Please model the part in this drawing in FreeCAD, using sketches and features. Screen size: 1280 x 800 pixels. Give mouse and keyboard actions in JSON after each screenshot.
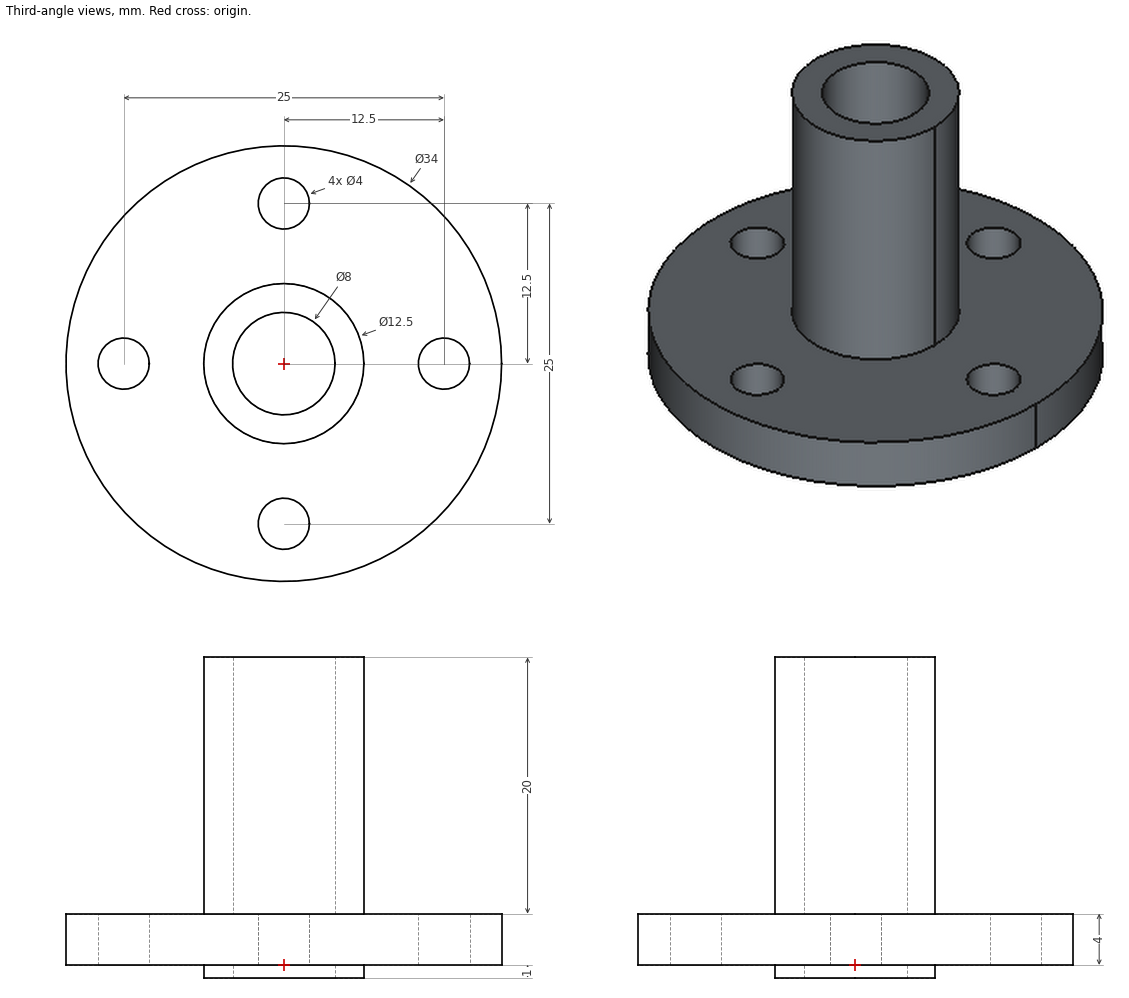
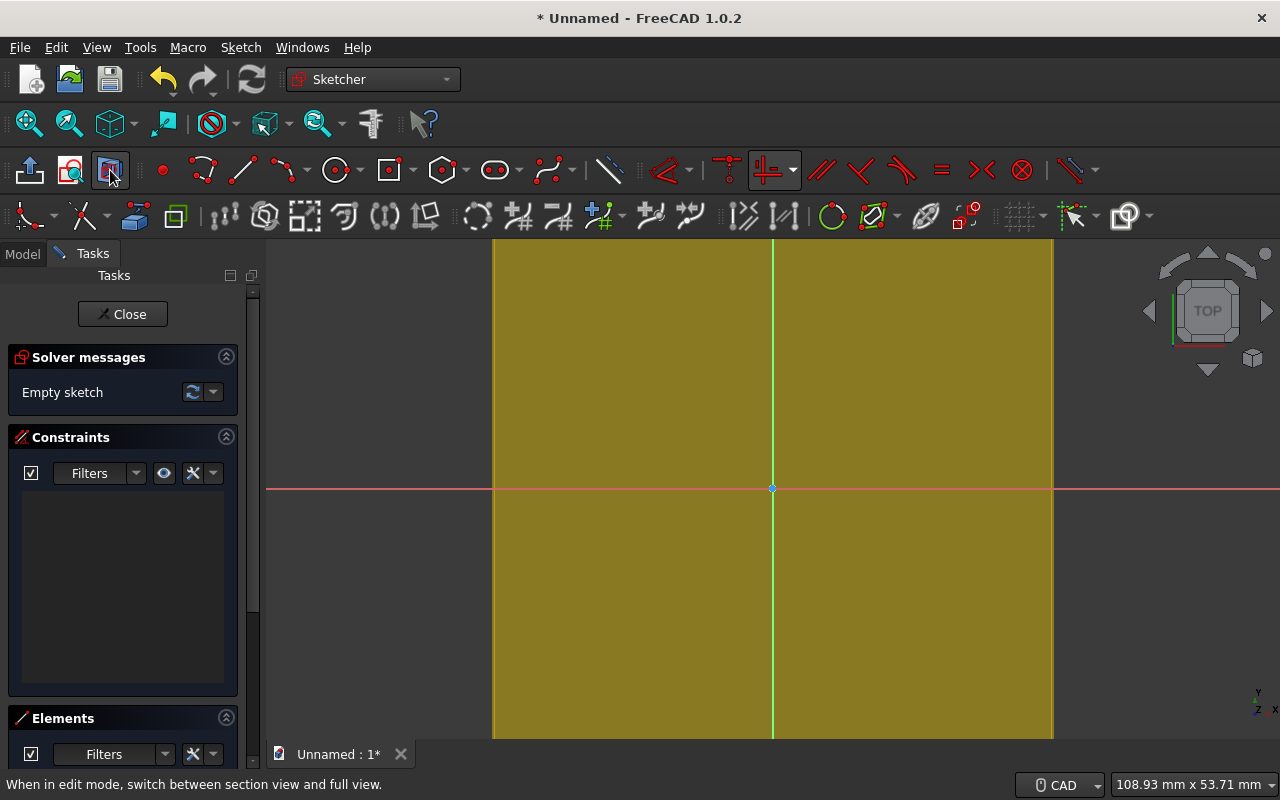
{"action": "scroll", "coordinate": [813, 489], "scroll_direction": "up", "scroll_amount": 5}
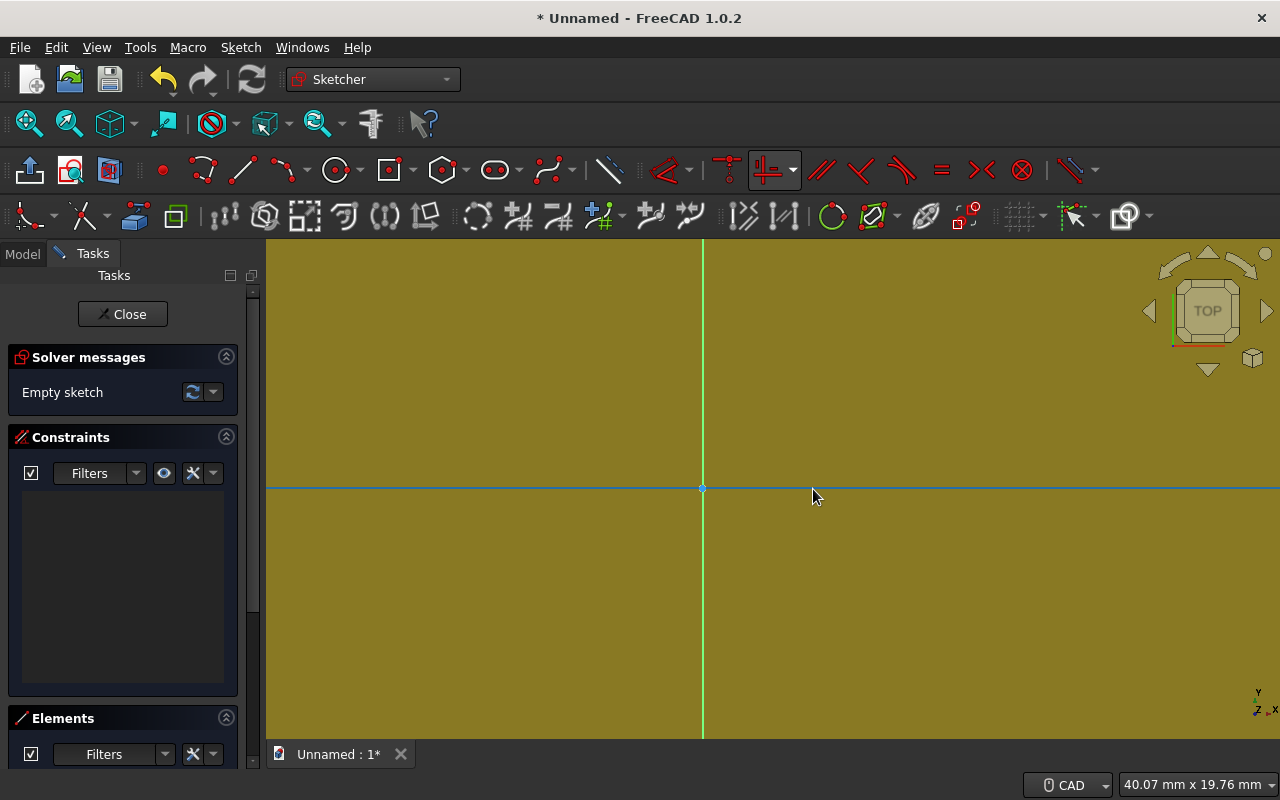
{"action": "left_click", "coordinate": [336, 170]}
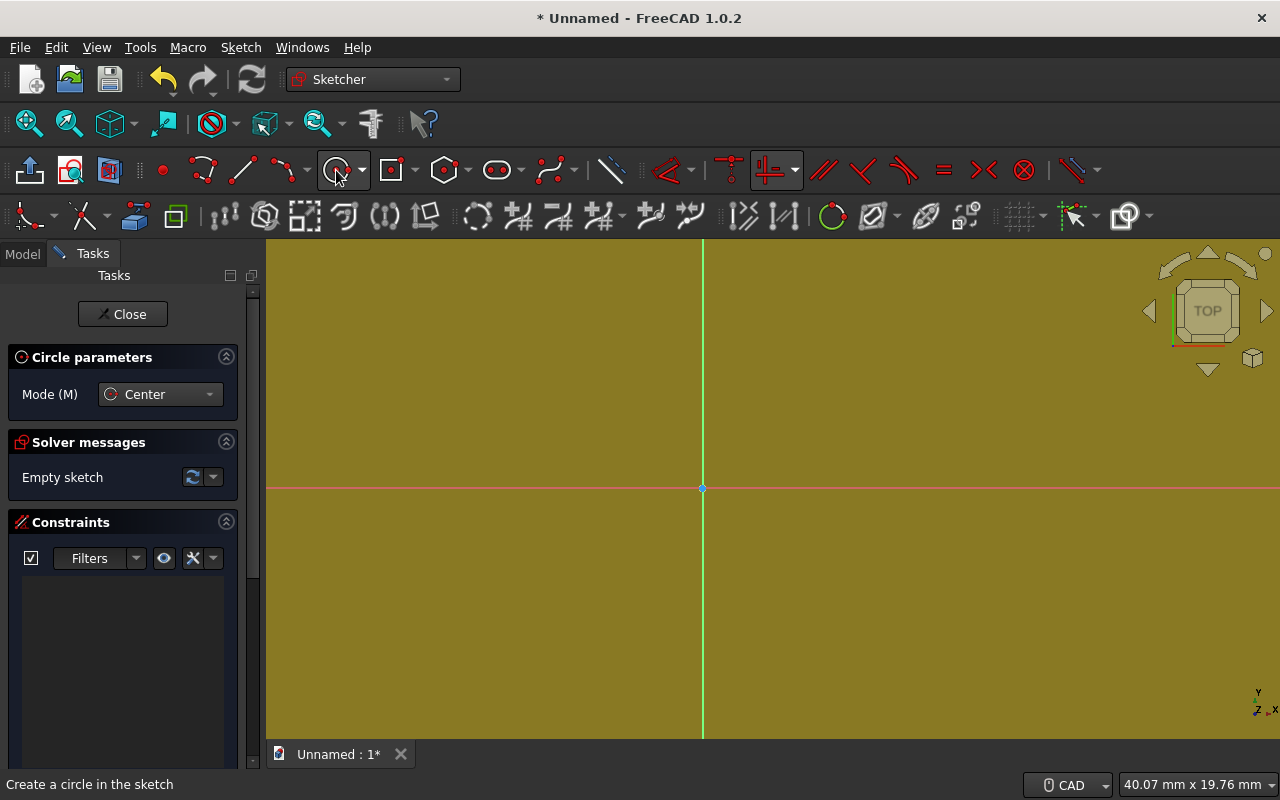
{"action": "left_click", "coordinate": [703, 488]}
{"action": "mouse_move", "coordinate": [815, 376]}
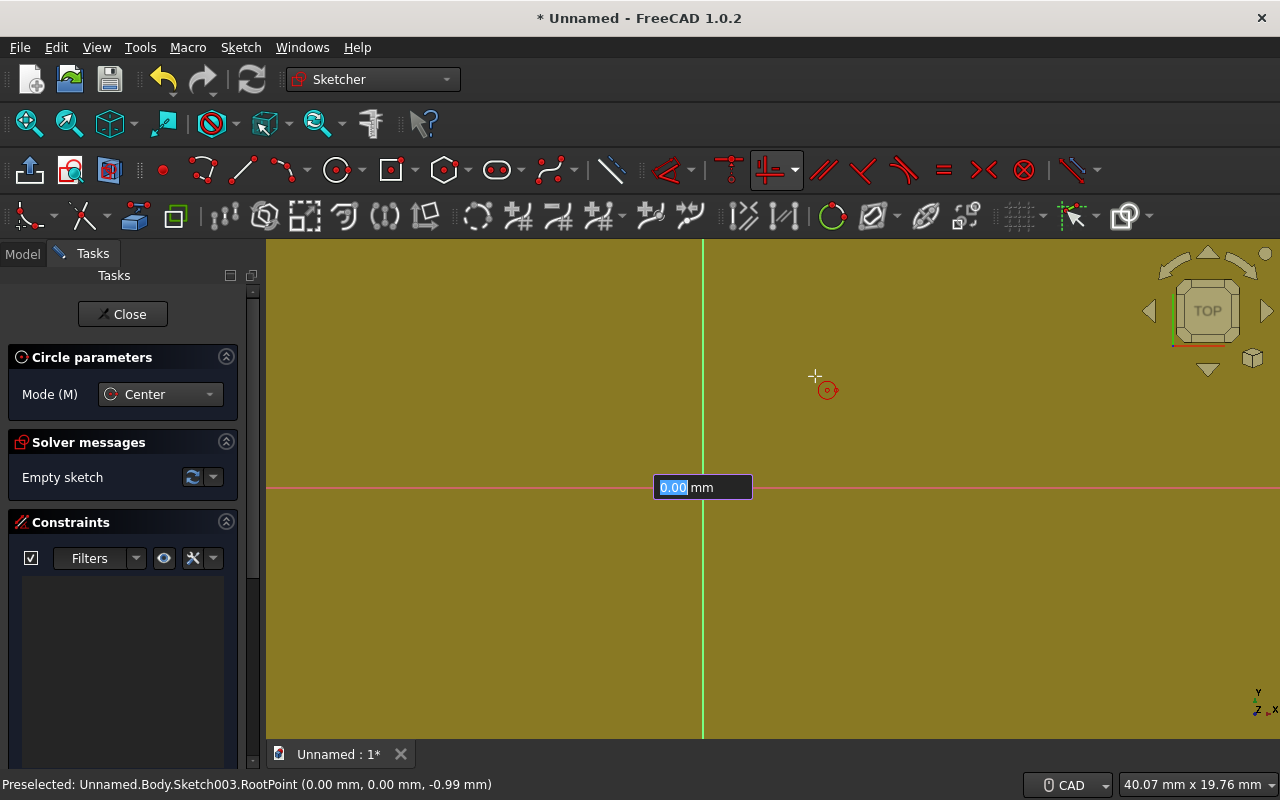
{"action": "type", "text": "12.5"}
{"action": "key", "text": "Return"}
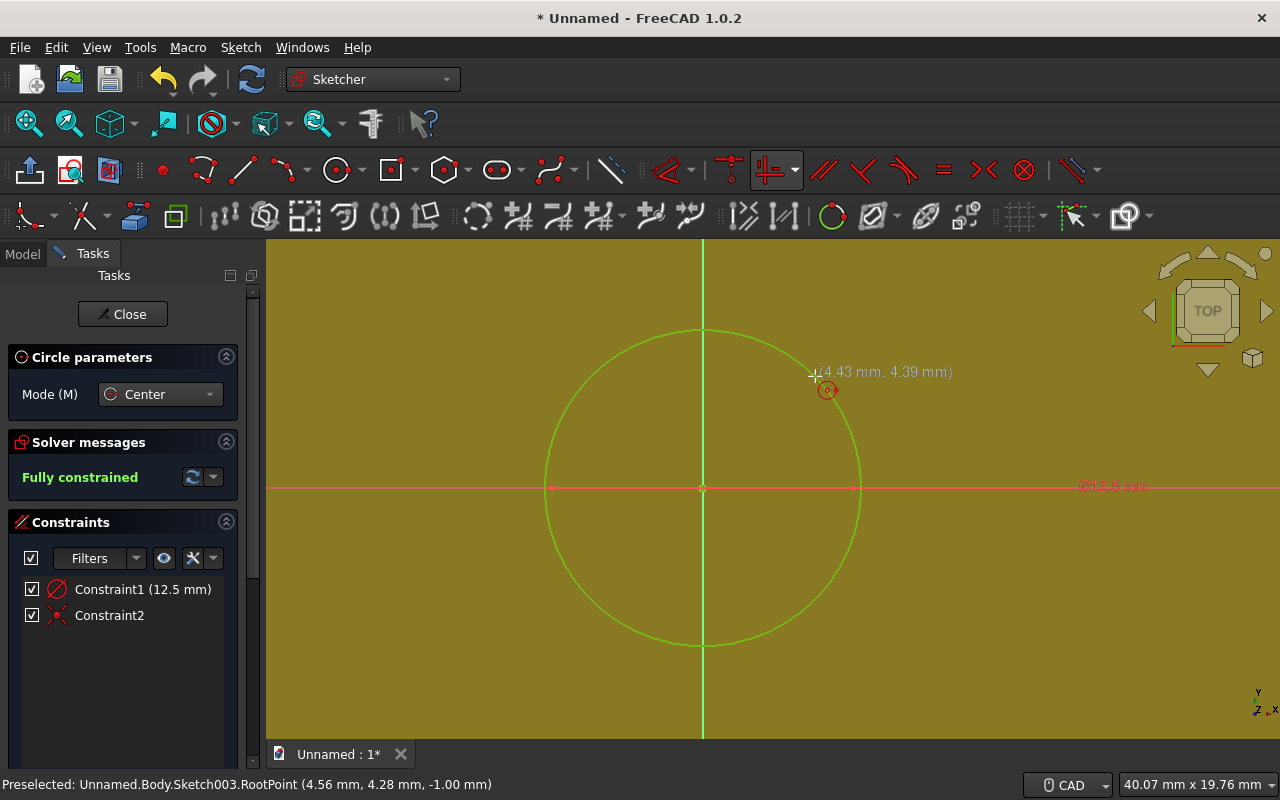
{"action": "left_click", "coordinate": [703, 488]}
{"action": "mouse_move", "coordinate": [775, 417]}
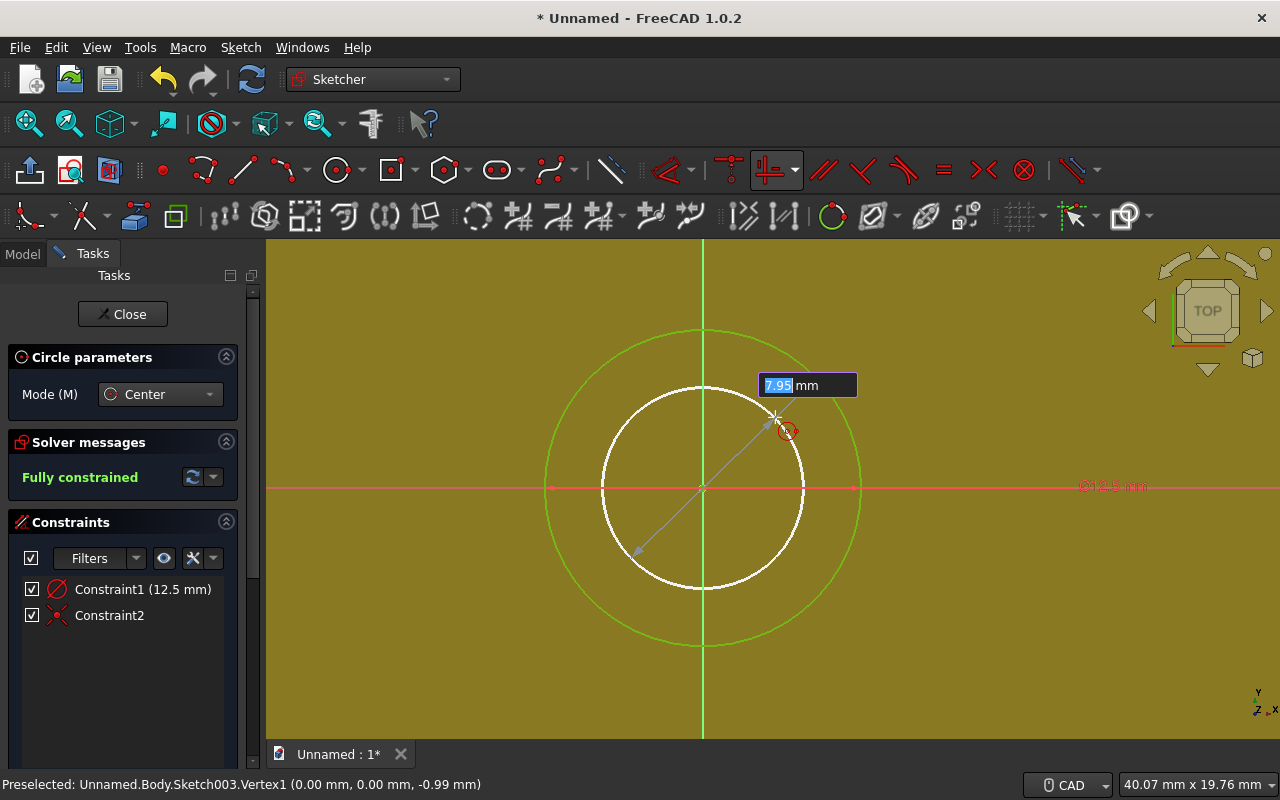
{"action": "type", "text": "8"}
{"action": "key", "text": "Return"}
{"action": "key", "text": "Escape"}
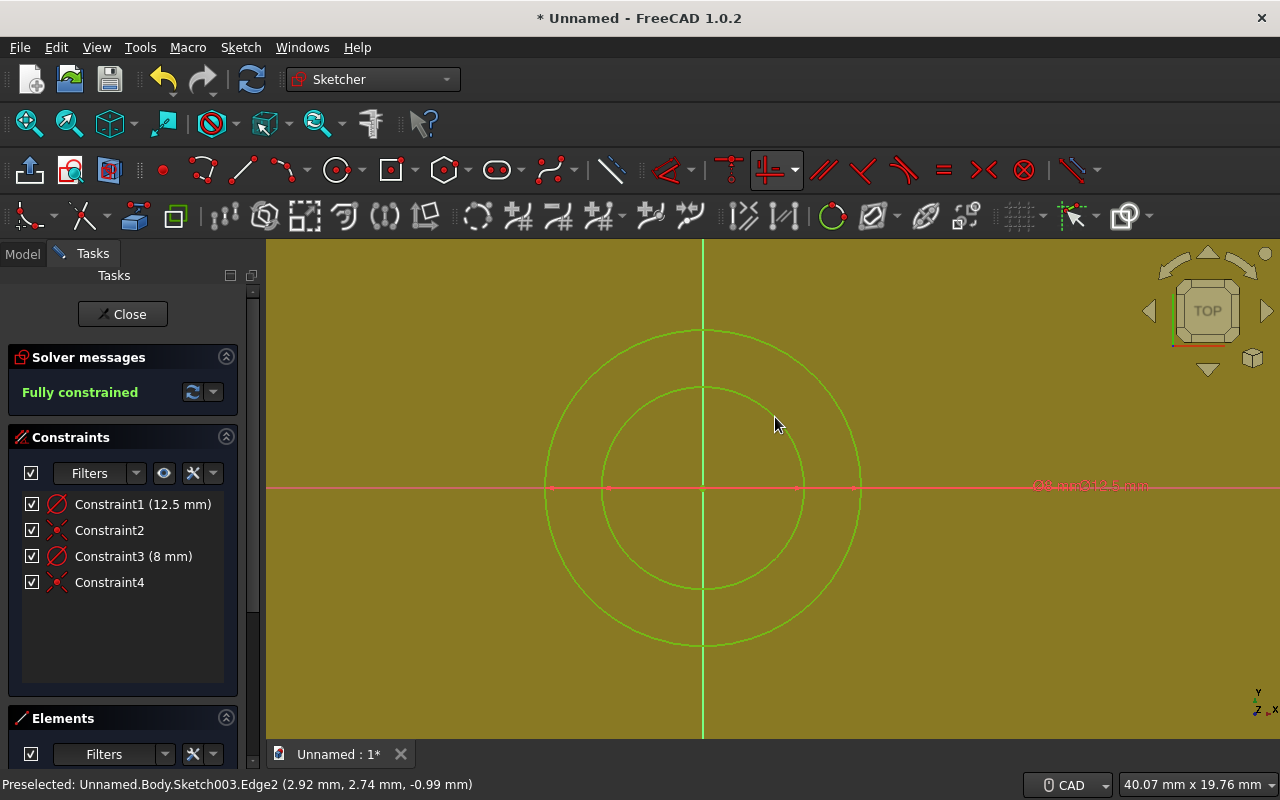
{"action": "left_click", "coordinate": [123, 314]}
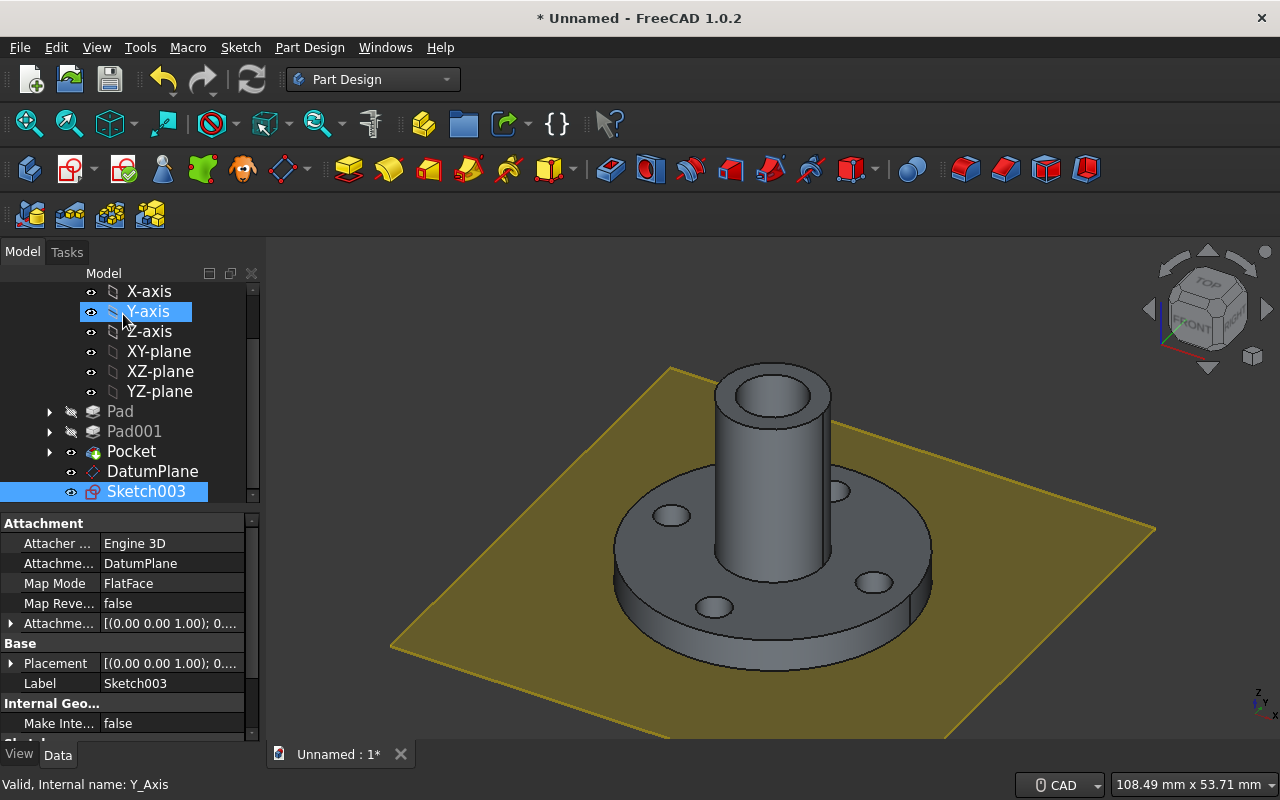
{"action": "left_click", "coordinate": [350, 170]}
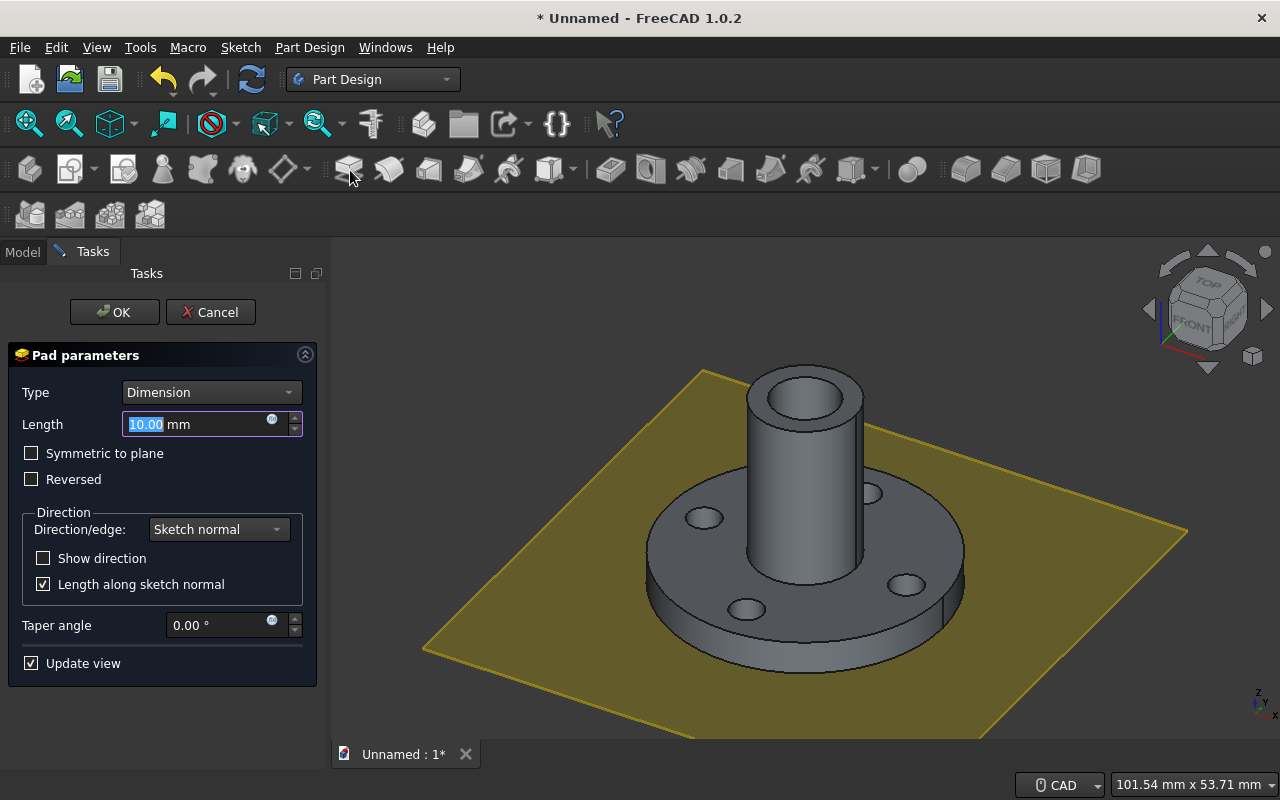
{"action": "type", "text": "1"}
{"action": "key", "text": "Tab"}